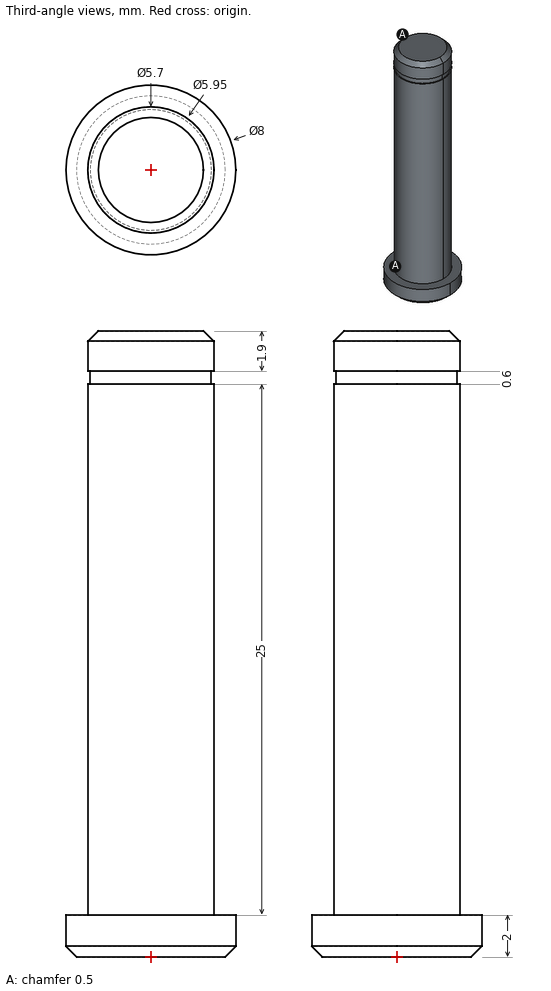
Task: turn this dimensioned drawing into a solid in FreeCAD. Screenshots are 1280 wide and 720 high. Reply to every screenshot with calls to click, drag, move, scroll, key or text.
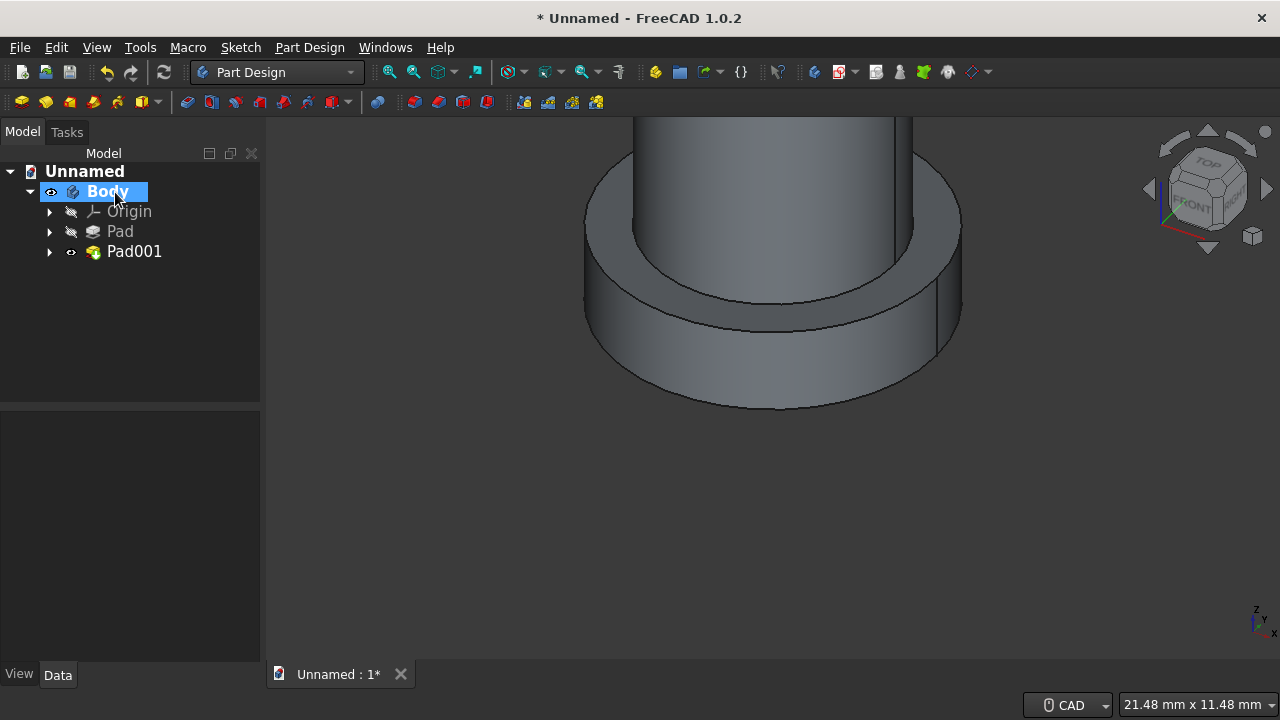
click(390, 72)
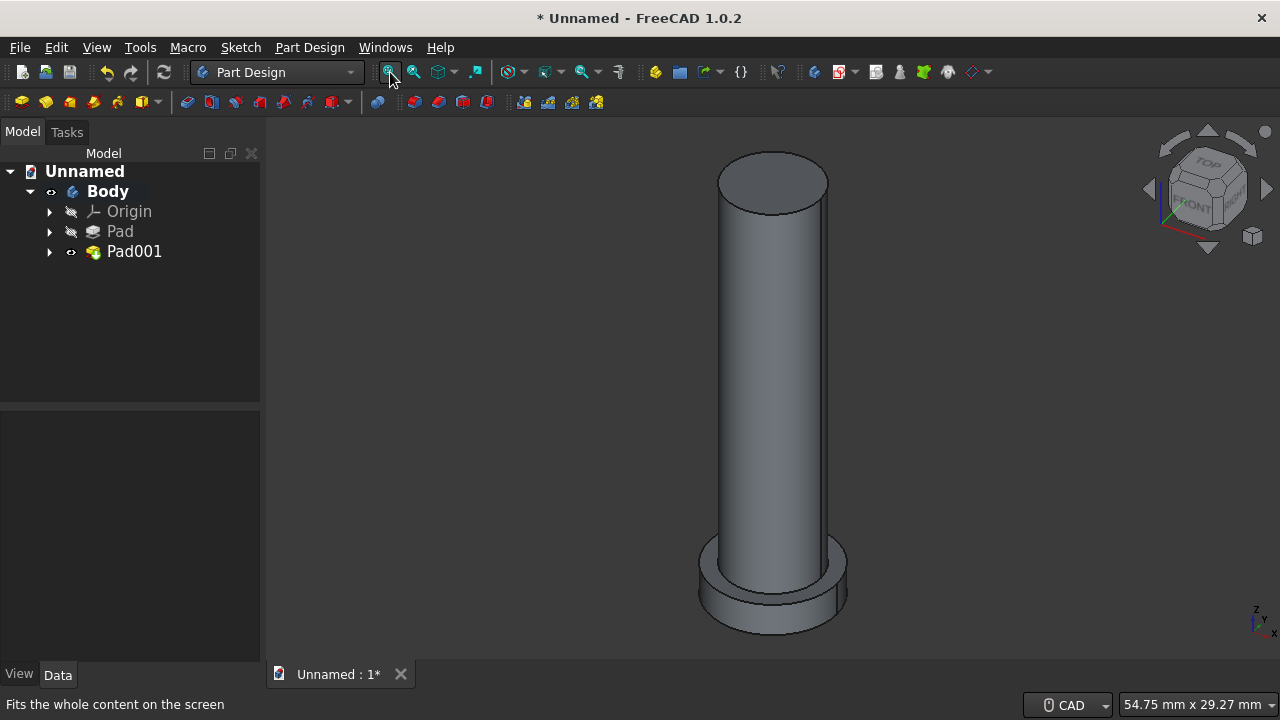
click(773, 182)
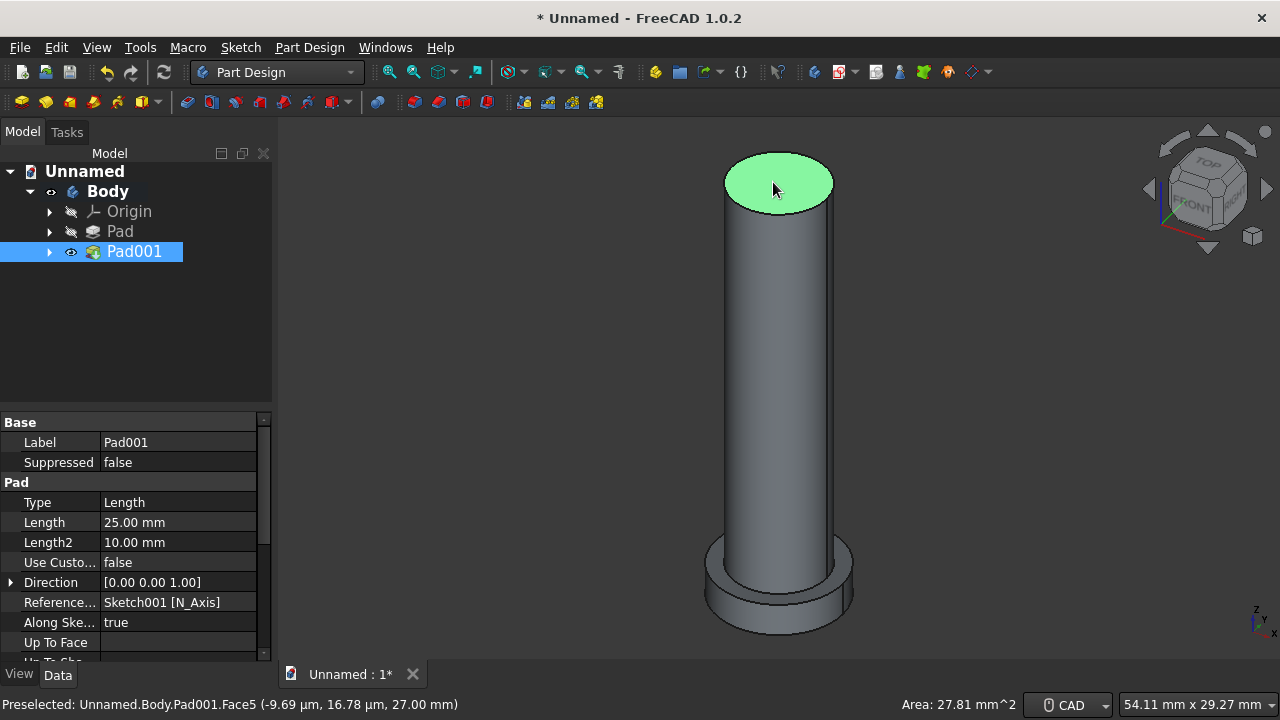
click(840, 72)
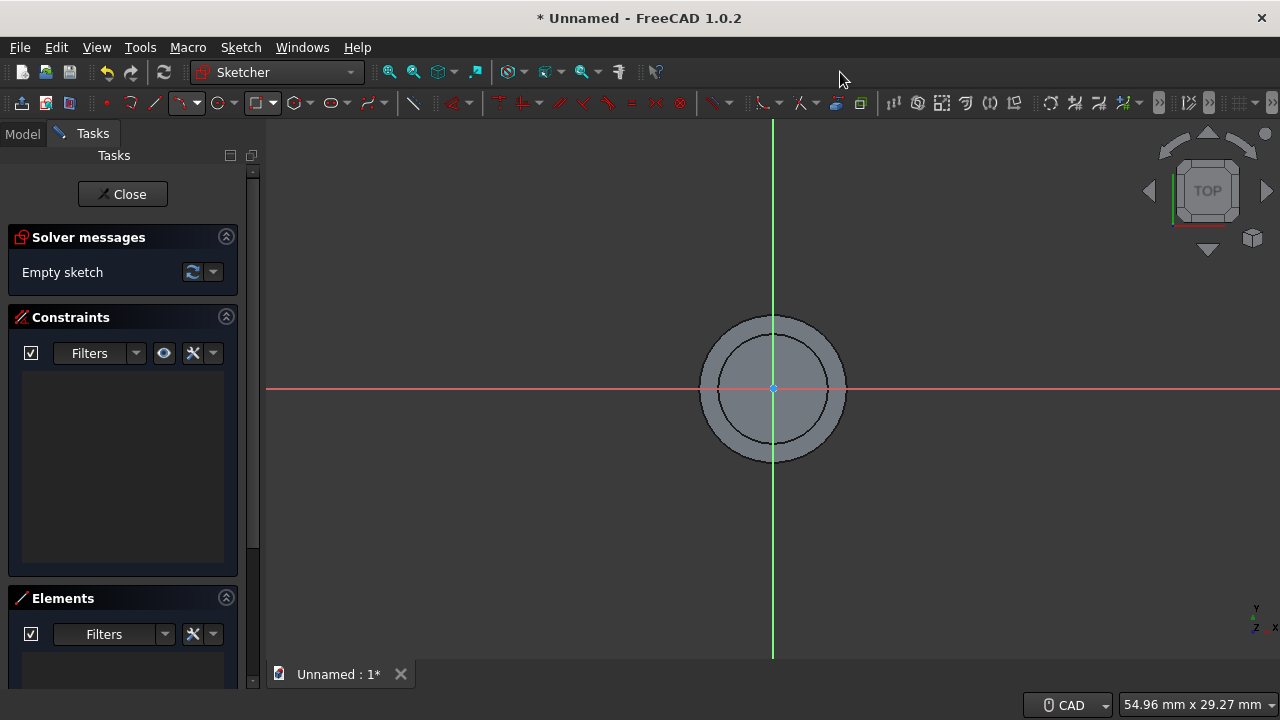
scroll(803, 389, up, 6)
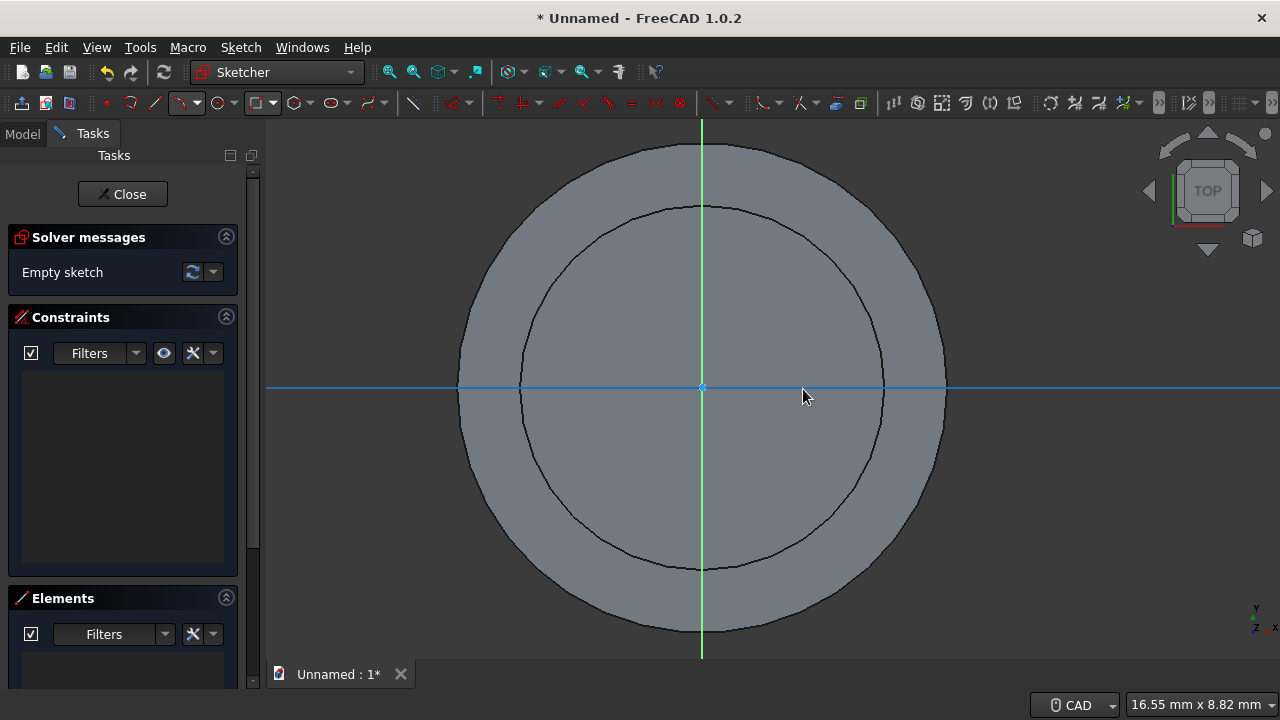
click(218, 104)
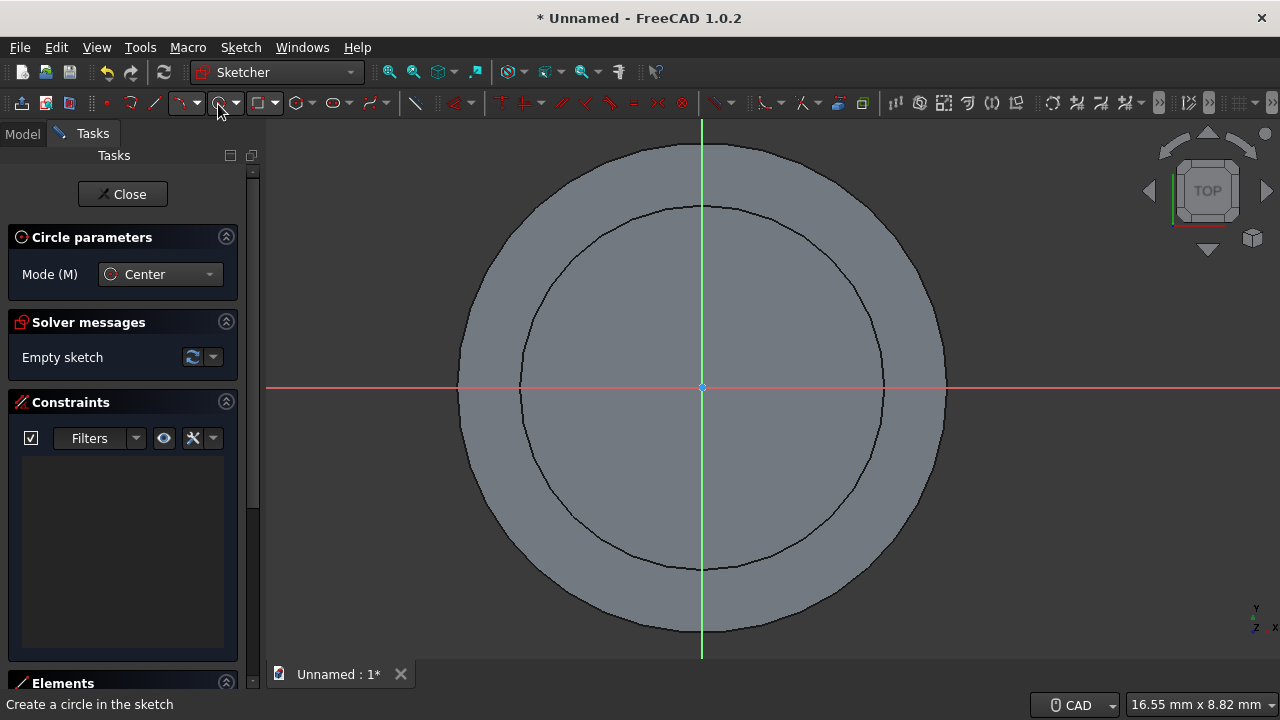
click(702, 388)
move(826, 264)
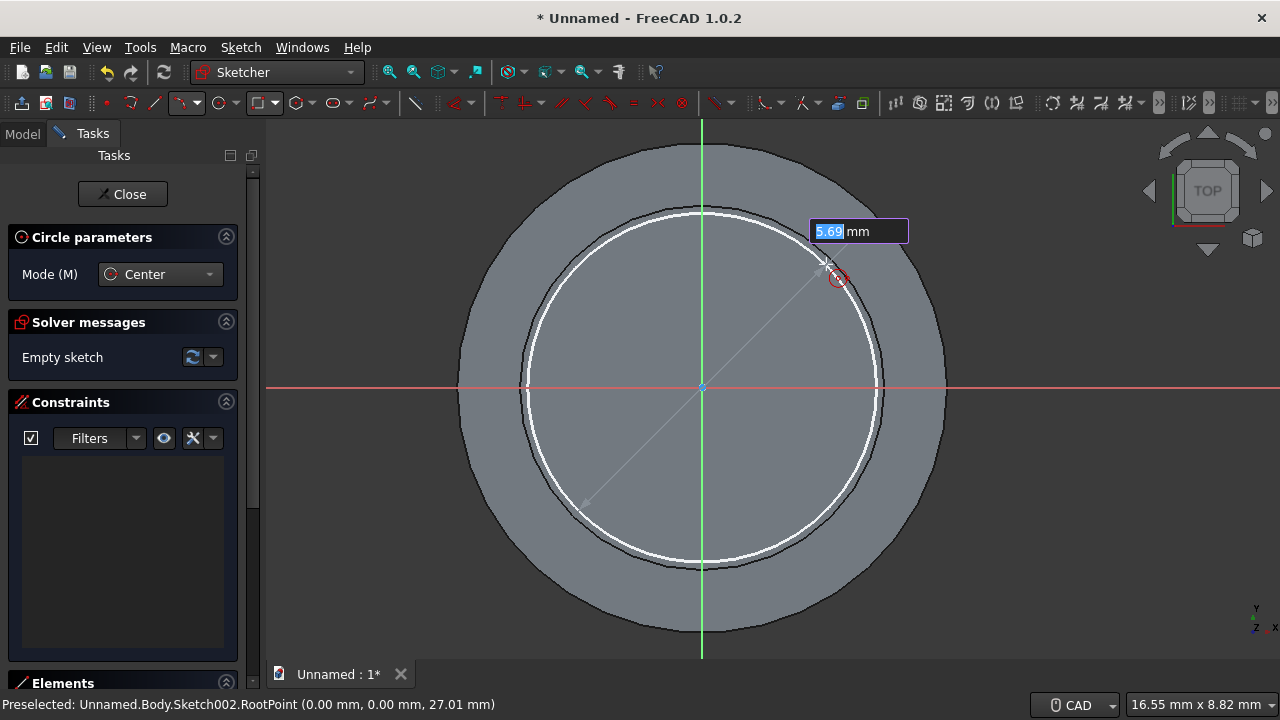
text(5.7)
key(Return)
key(Escape)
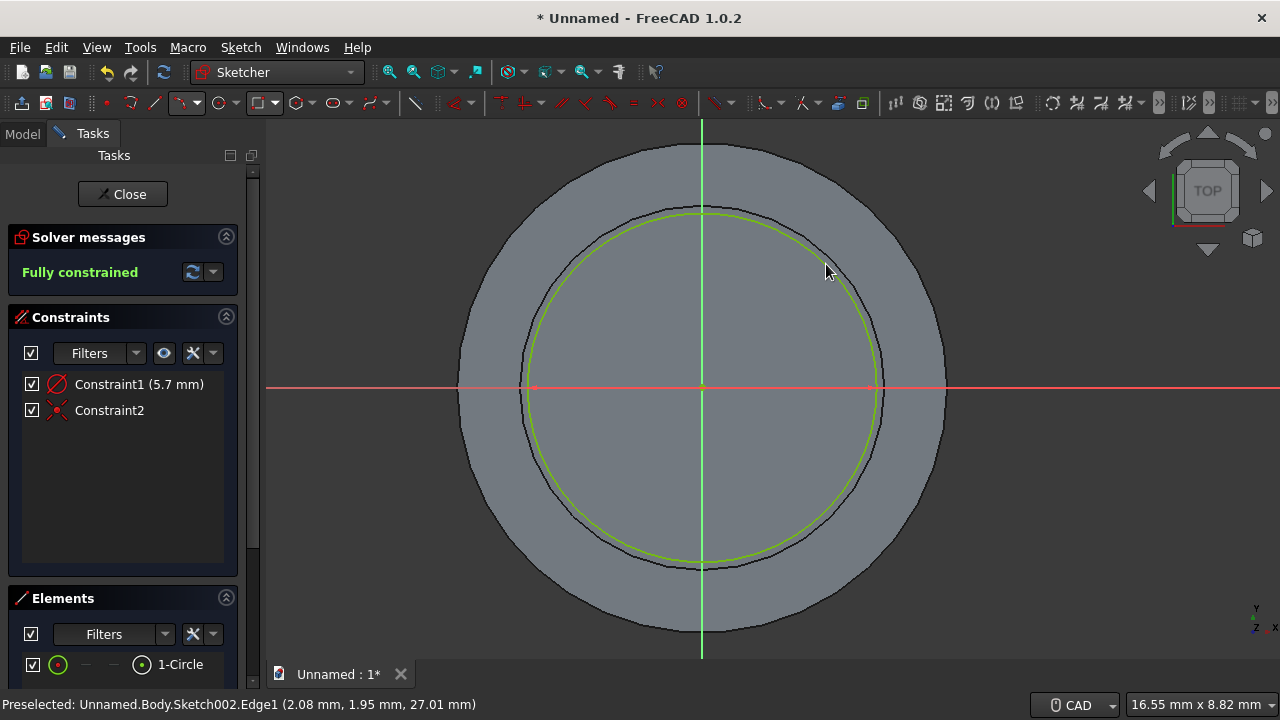
click(123, 194)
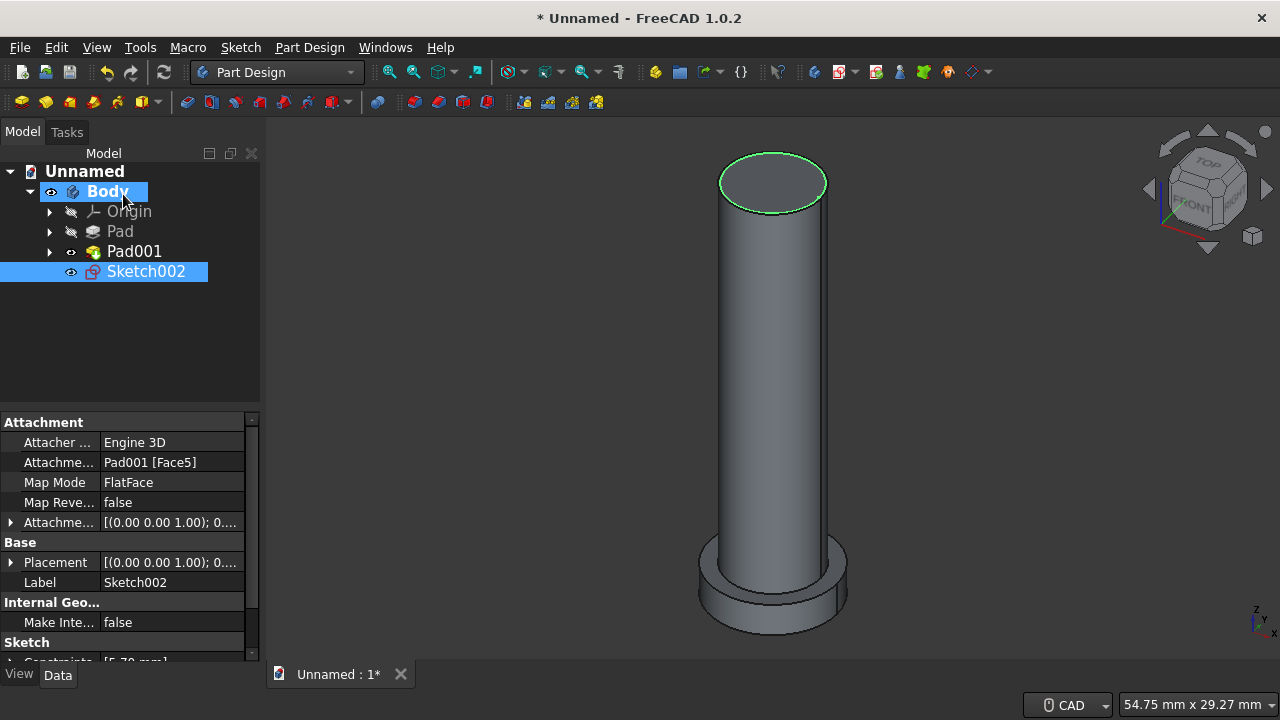
click(22, 102)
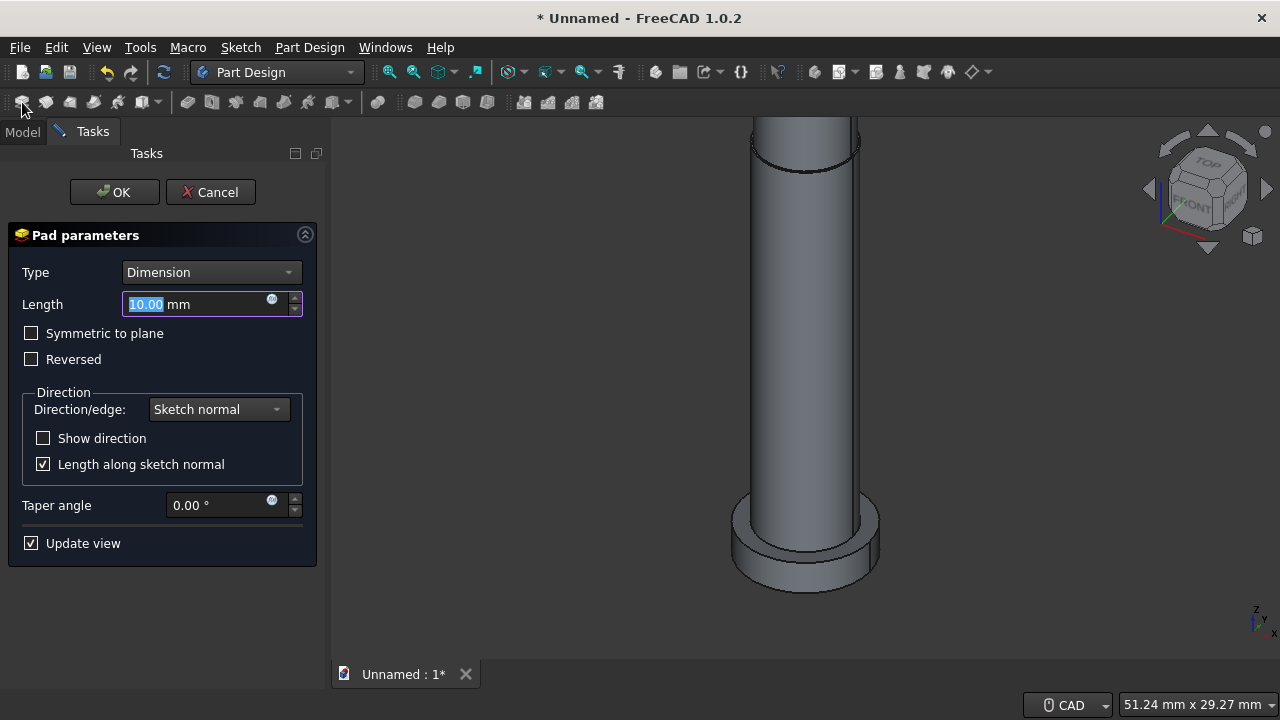
text(0.6)
key(Tab)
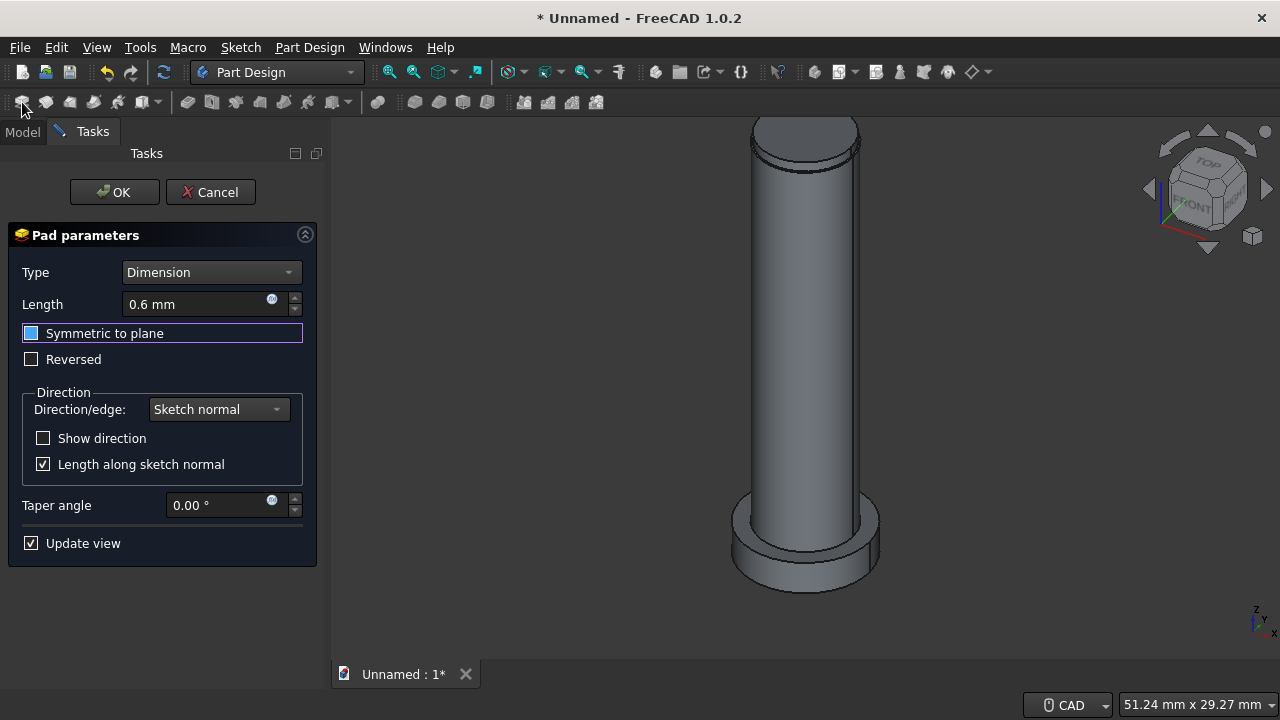
click(115, 192)